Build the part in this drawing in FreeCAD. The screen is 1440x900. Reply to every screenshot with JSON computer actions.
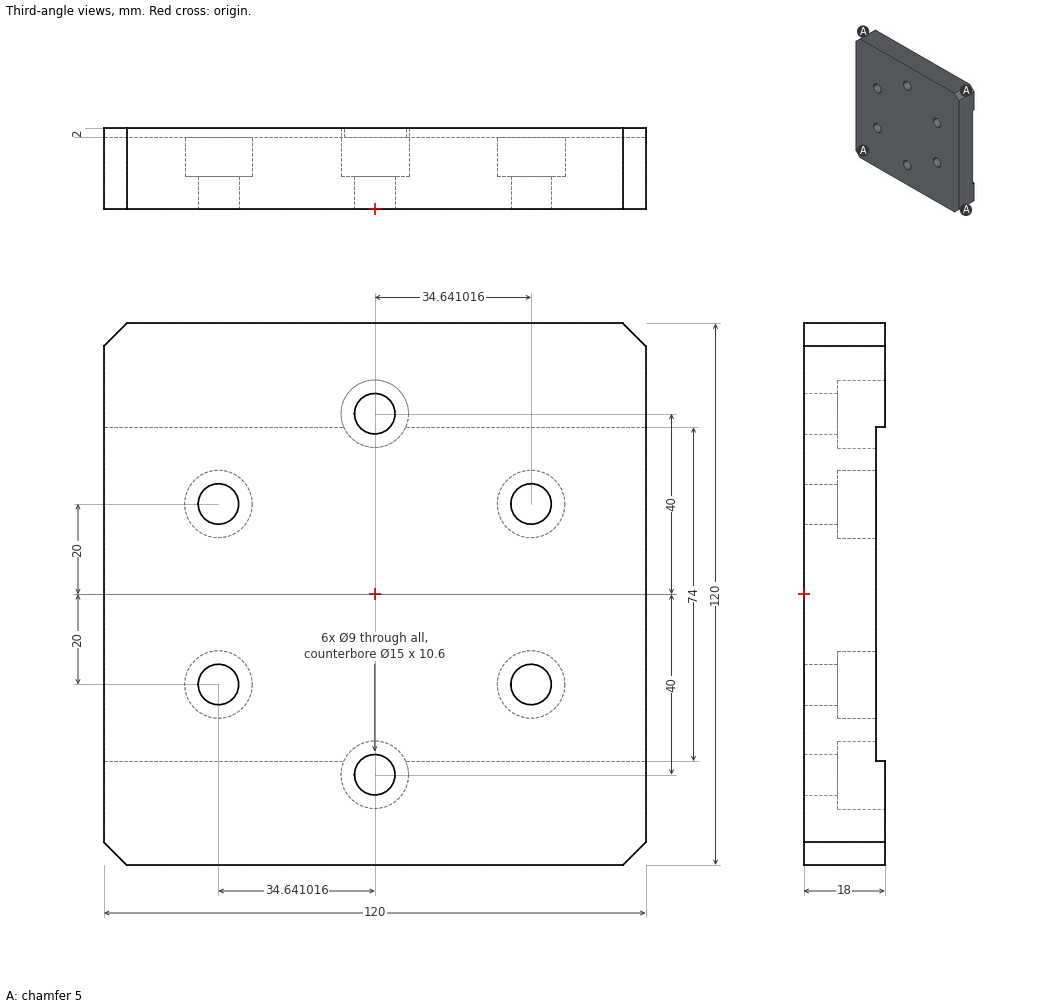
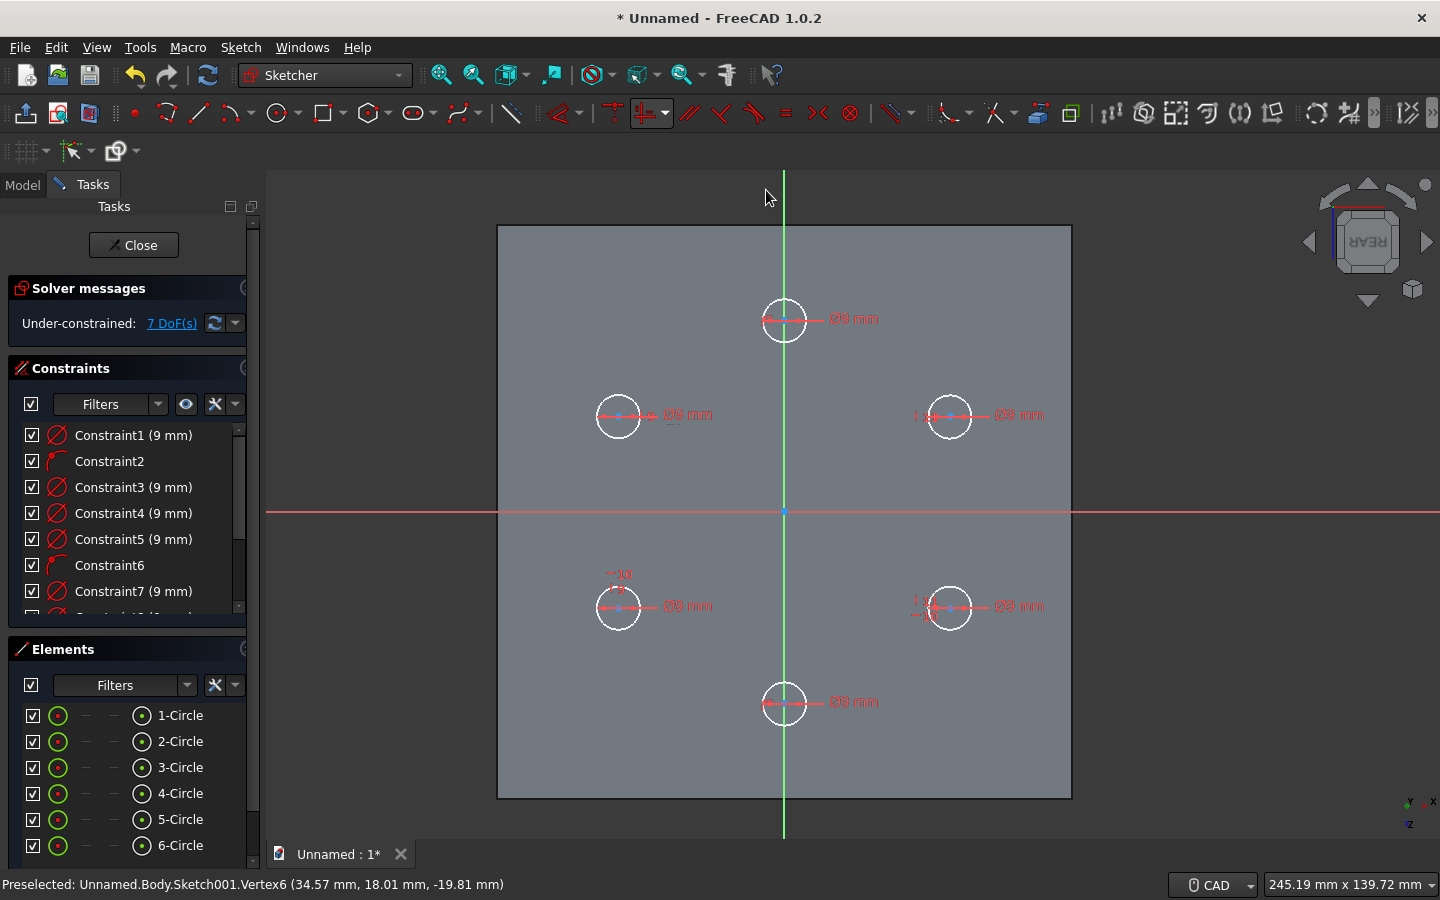
{"action": "left_click", "coordinate": [618, 417]}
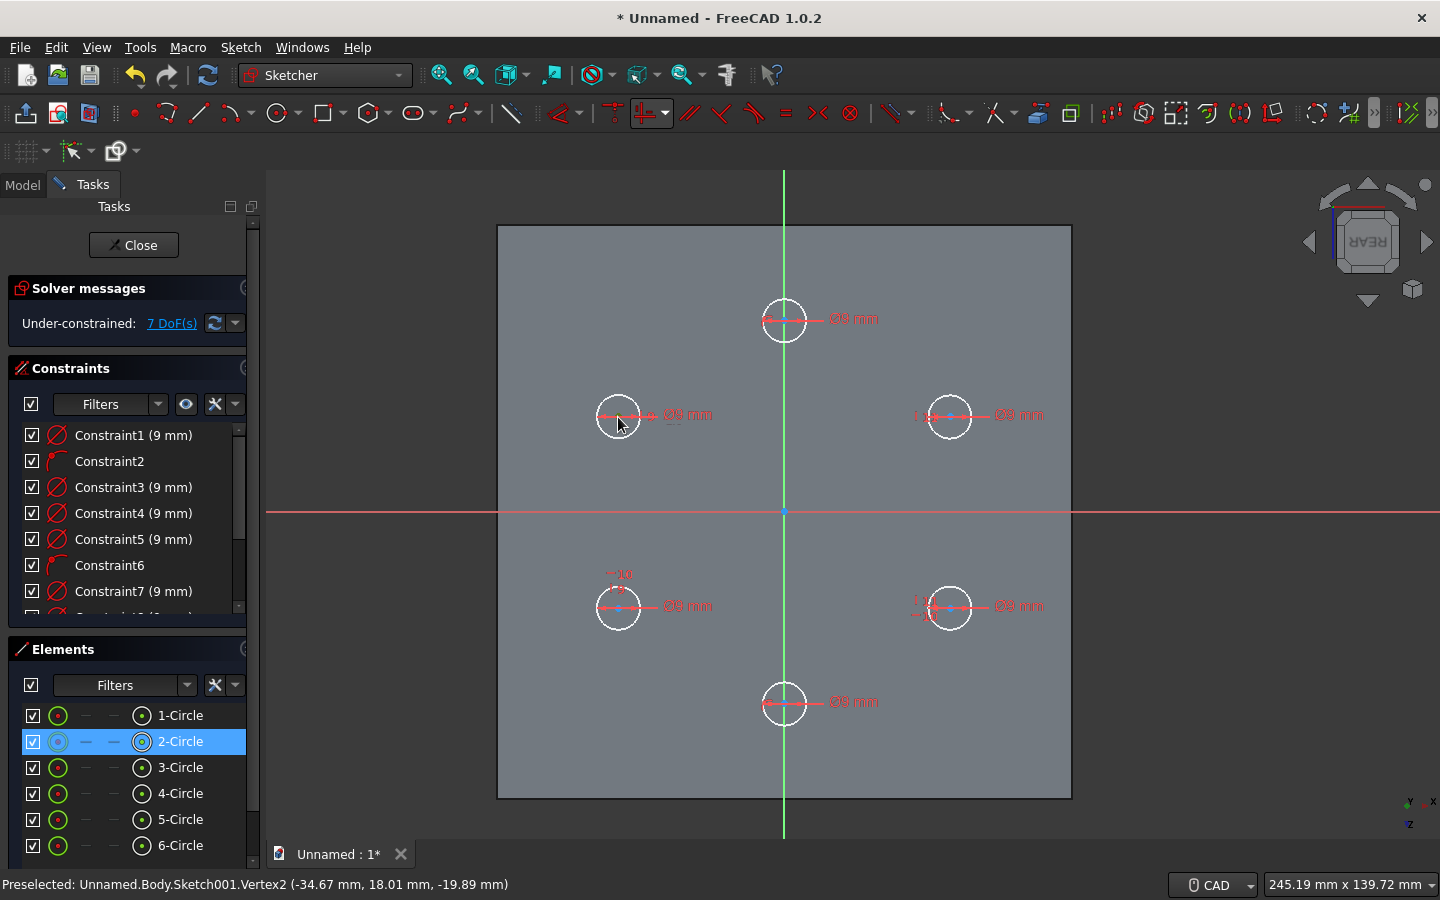
{"action": "left_click", "coordinate": [950, 417]}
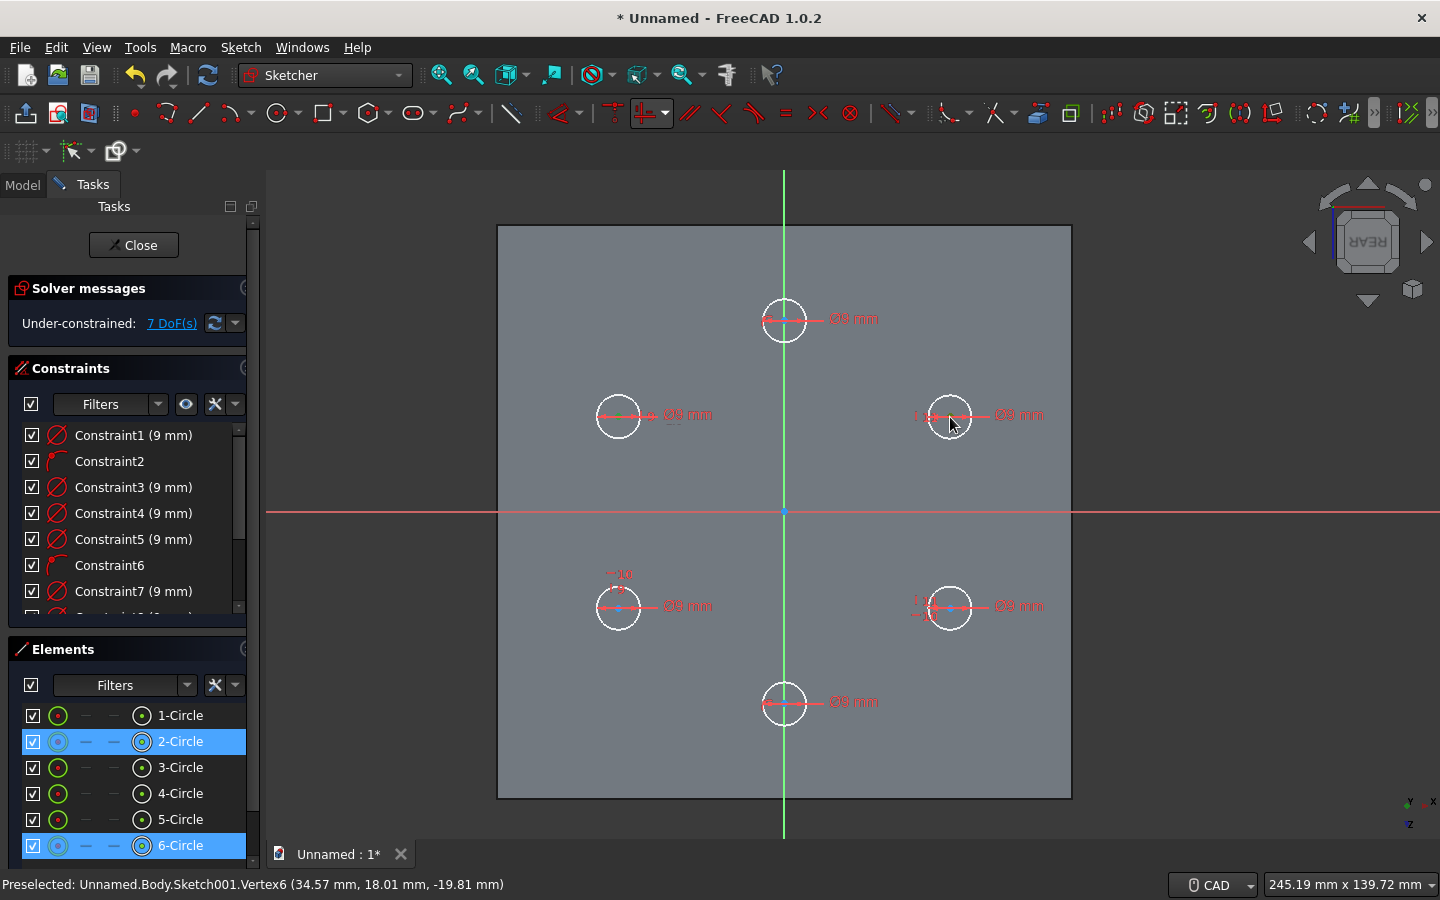
{"action": "key", "text": "h"}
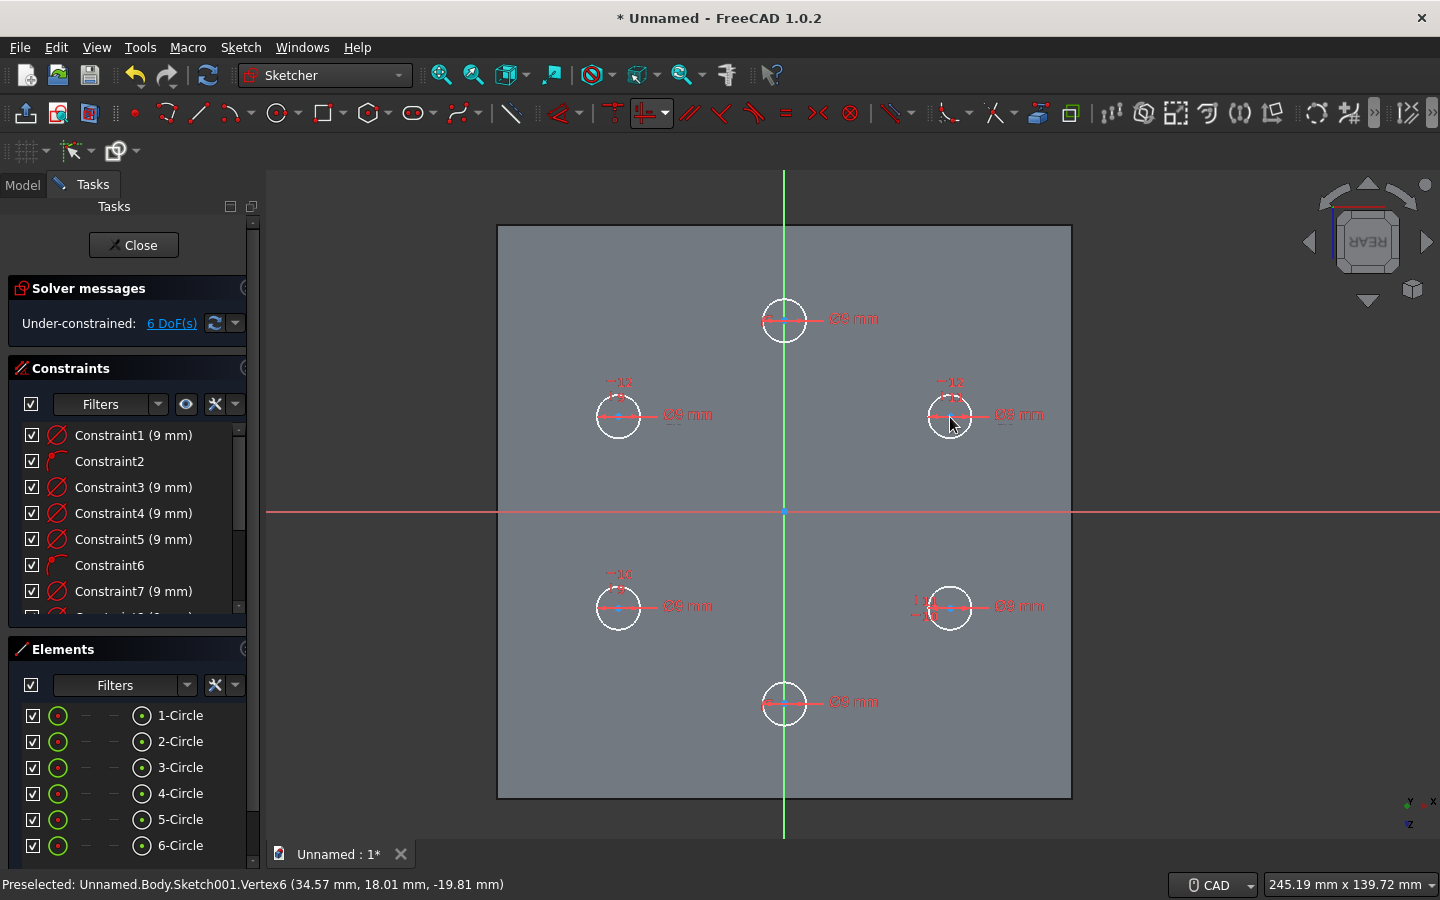
{"action": "left_click", "coordinate": [558, 114]}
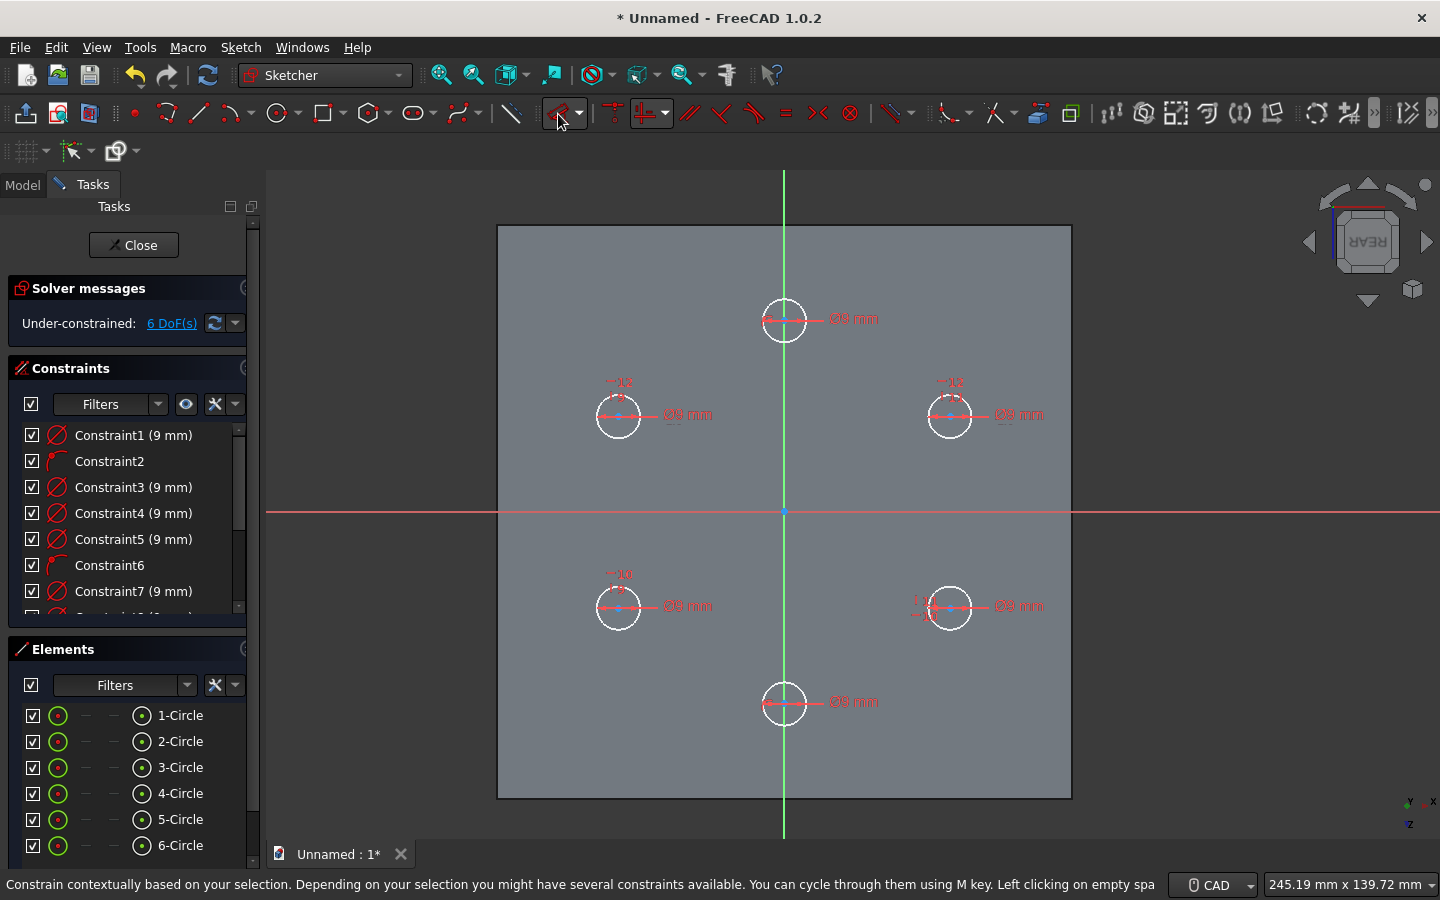
{"action": "left_click", "coordinate": [784, 321]}
{"action": "left_click", "coordinate": [818, 416]}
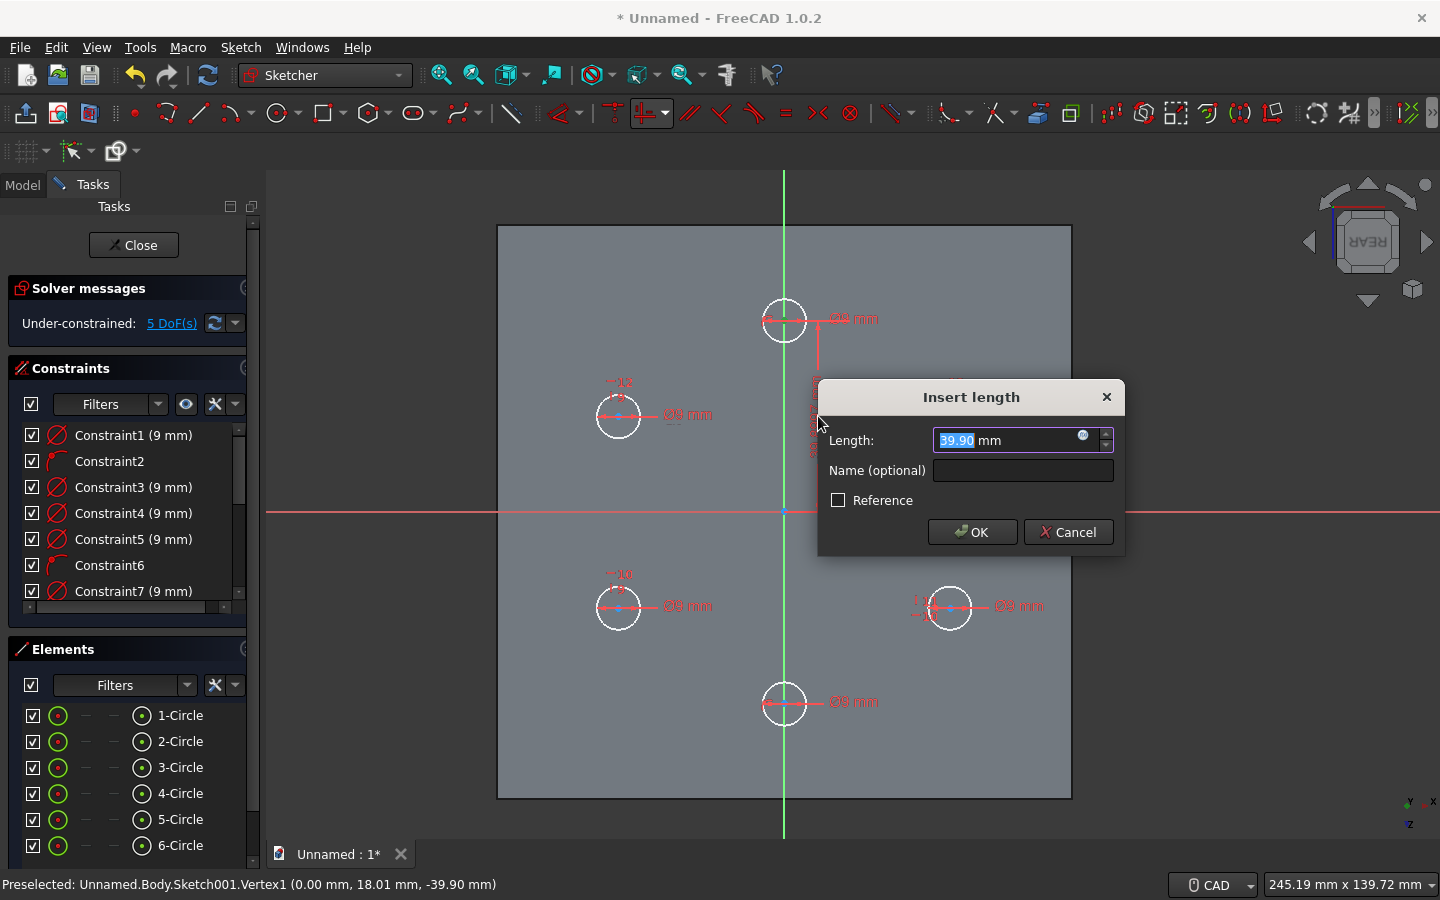
{"action": "type", "text": "40"}
{"action": "key", "text": "Return"}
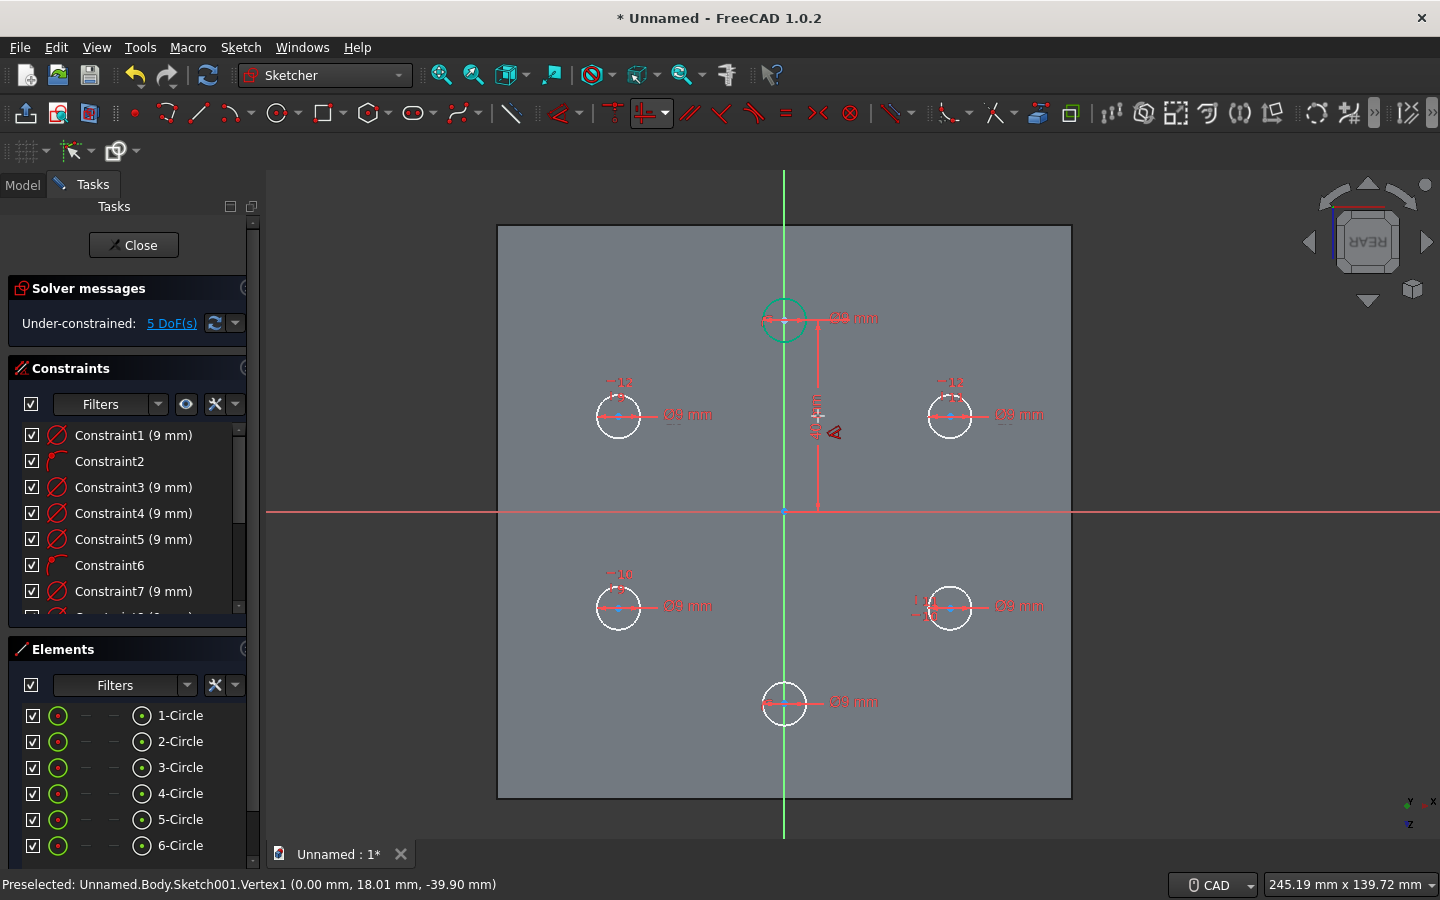
{"action": "left_click", "coordinate": [618, 417]}
{"action": "left_click", "coordinate": [584, 464]}